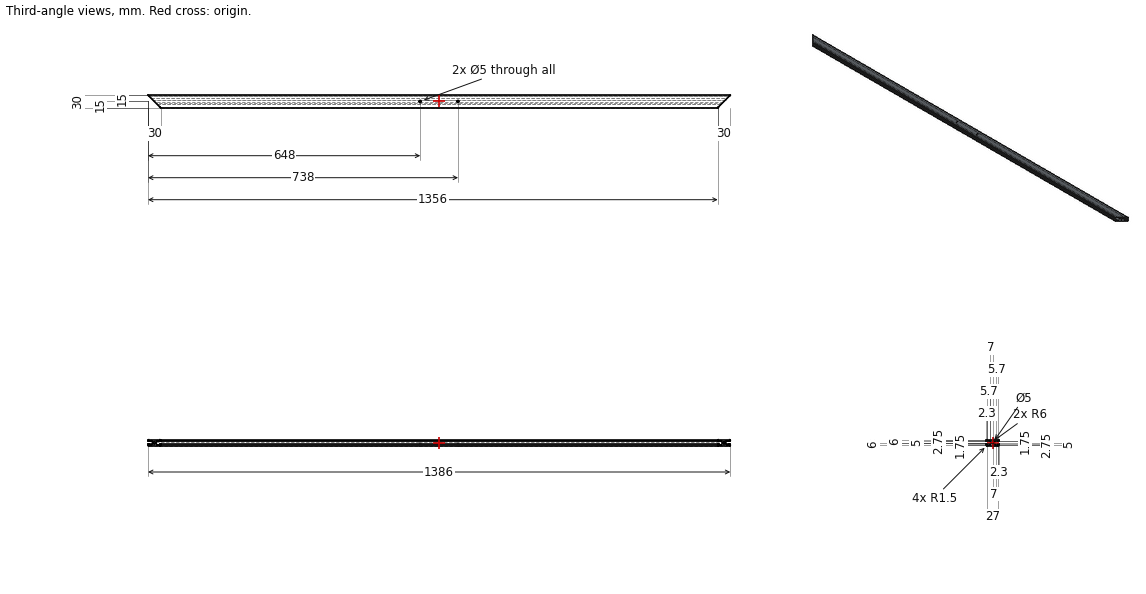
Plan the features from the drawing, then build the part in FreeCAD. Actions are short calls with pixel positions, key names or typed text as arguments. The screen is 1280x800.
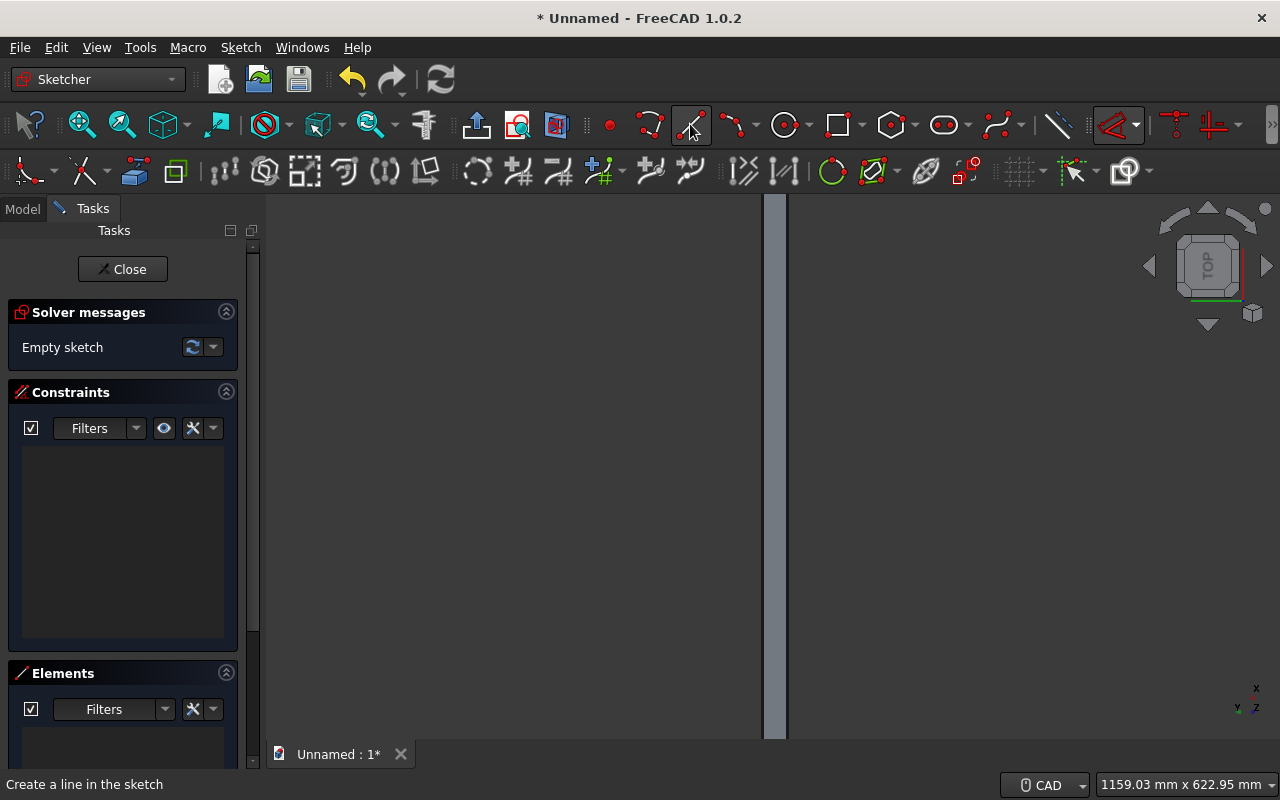
scroll(674, 467, down, 6)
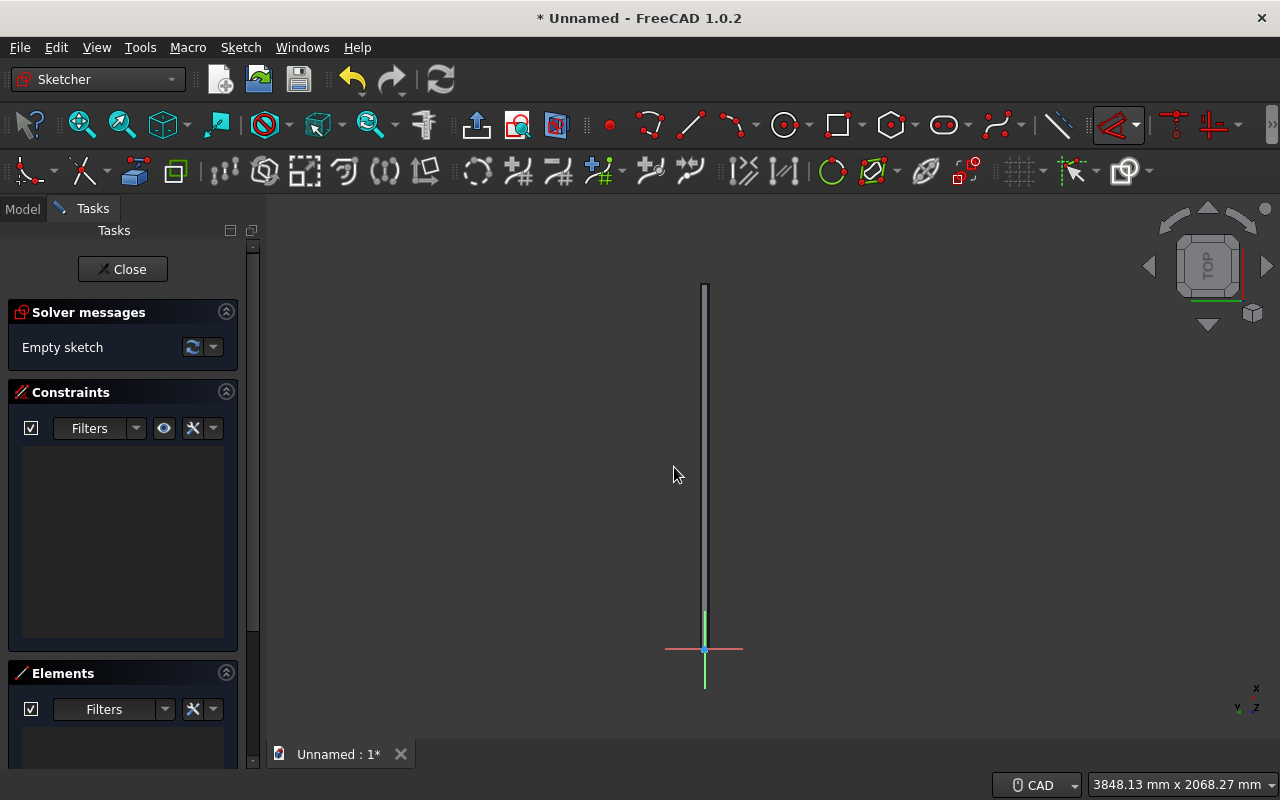
click(650, 126)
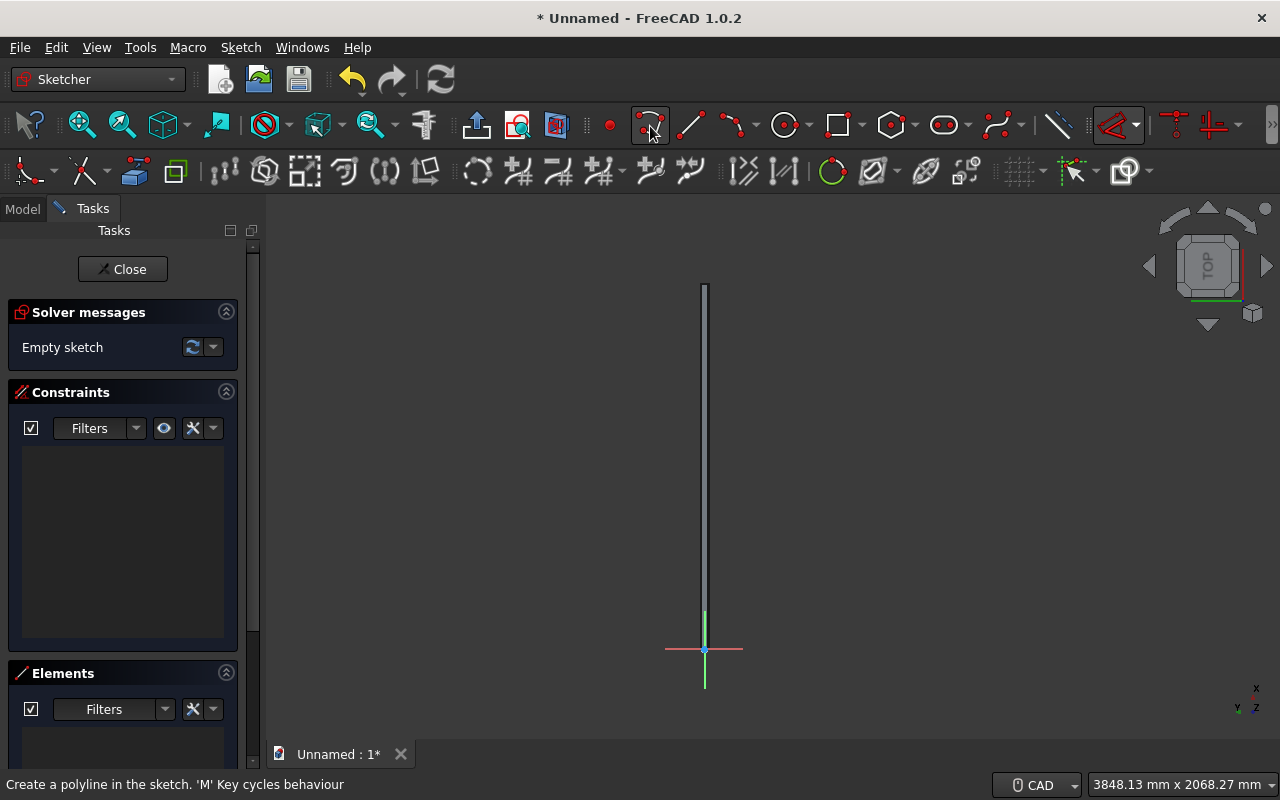
scroll(701, 649, up, 7)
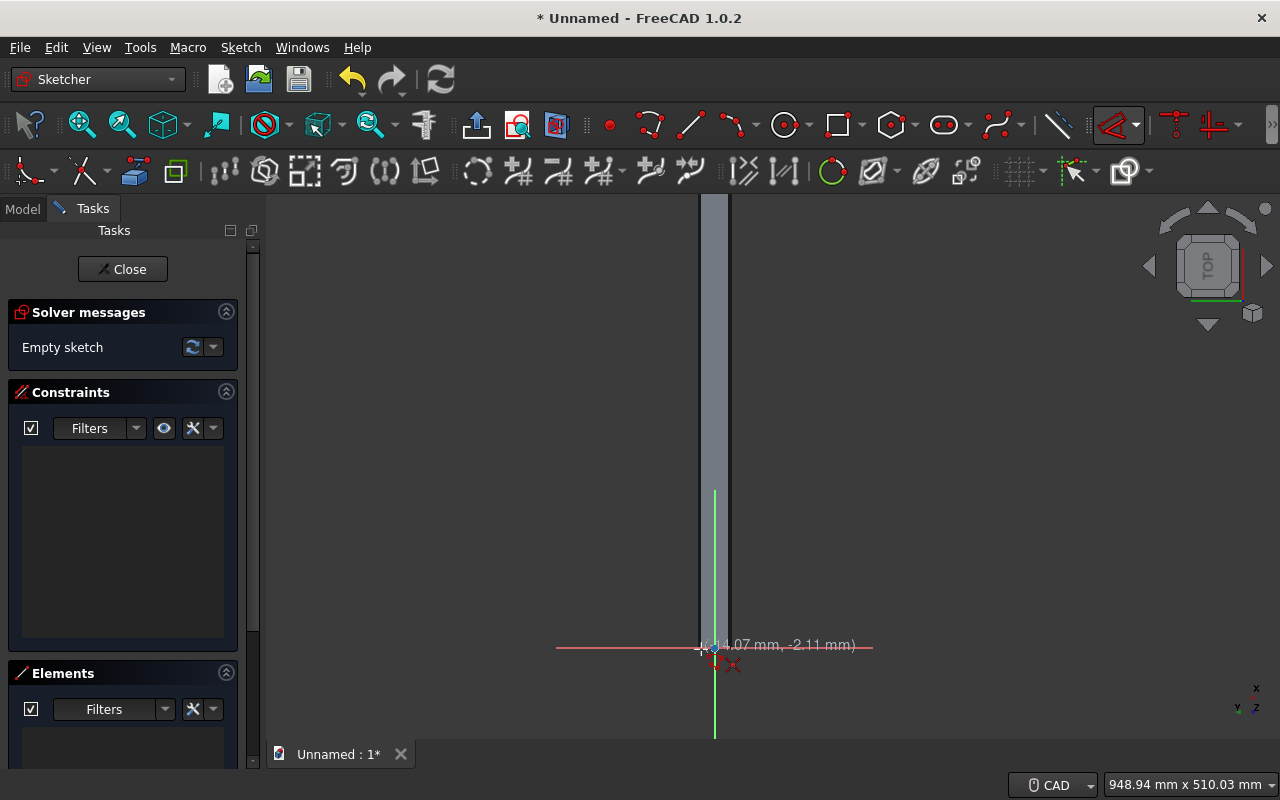
click(699, 648)
click(731, 639)
click(731, 616)
click(699, 648)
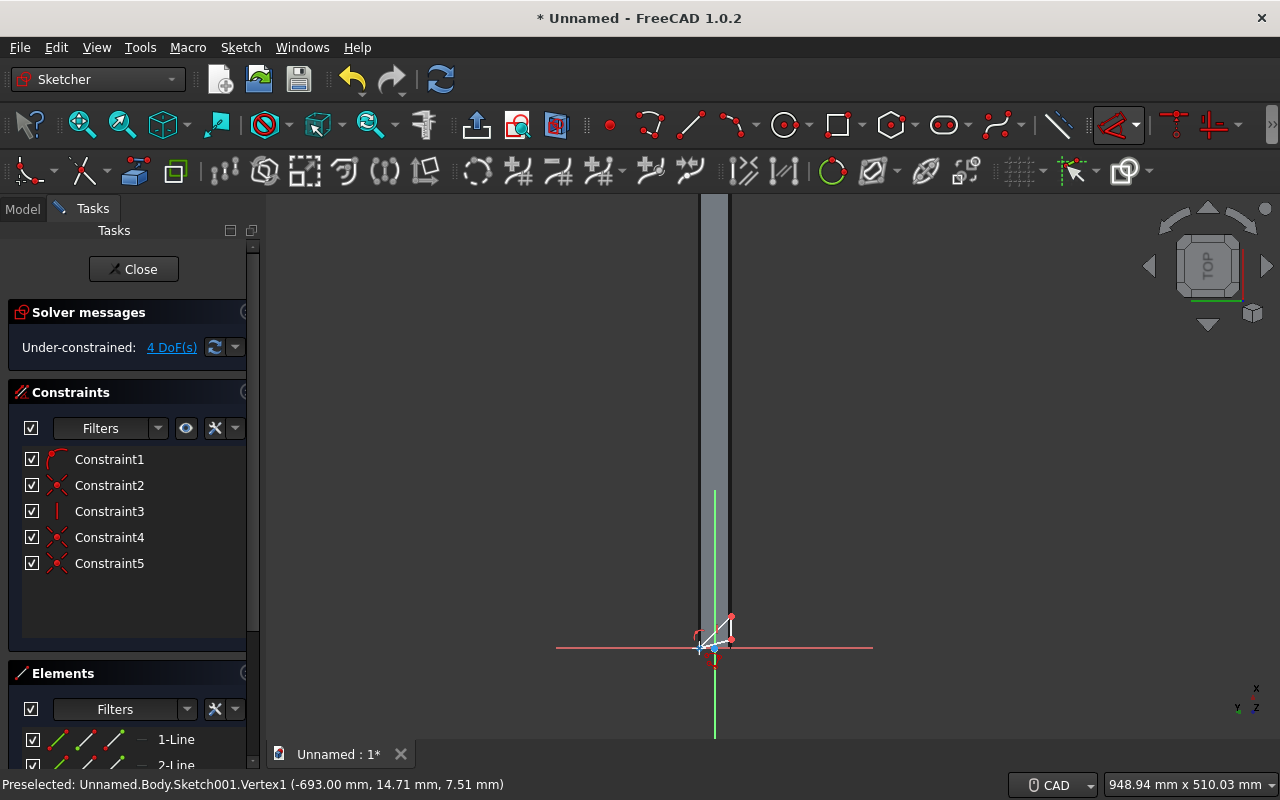
scroll(701, 649, down, 7)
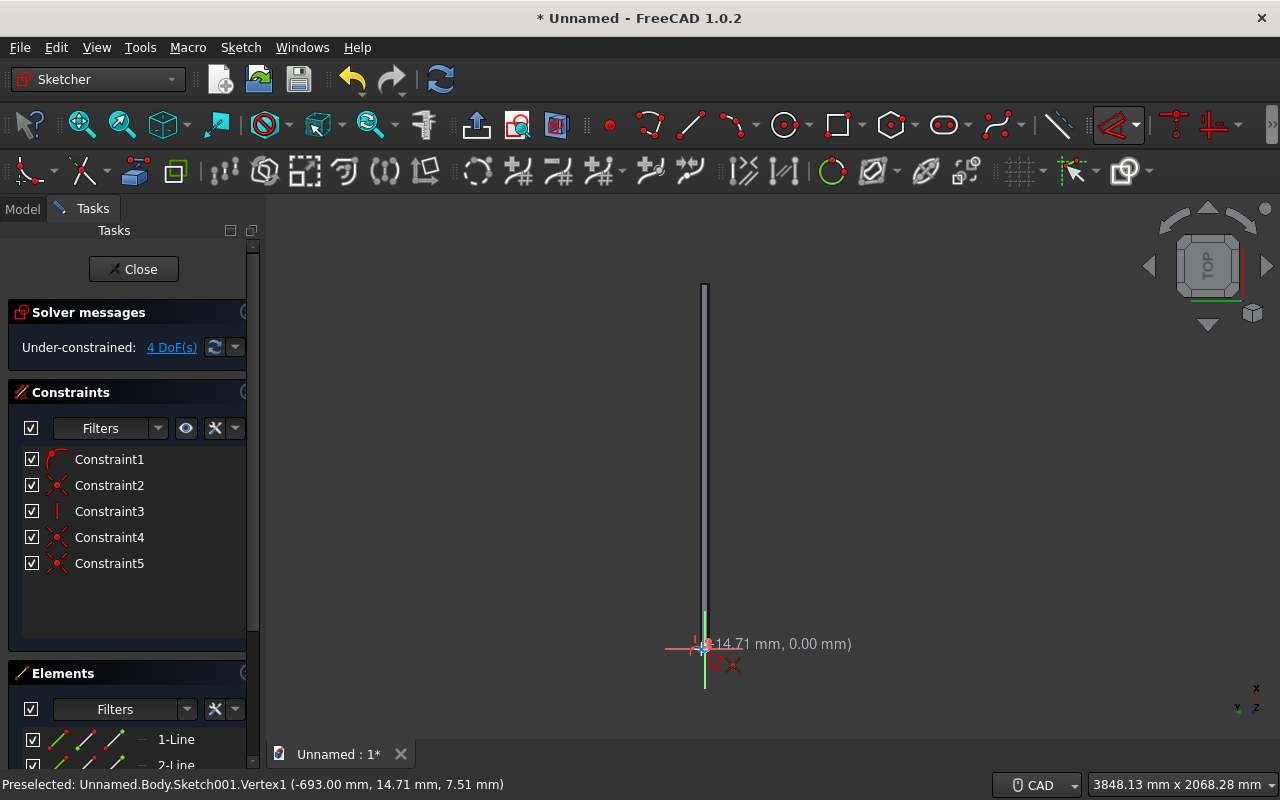
scroll(709, 292, up, 7)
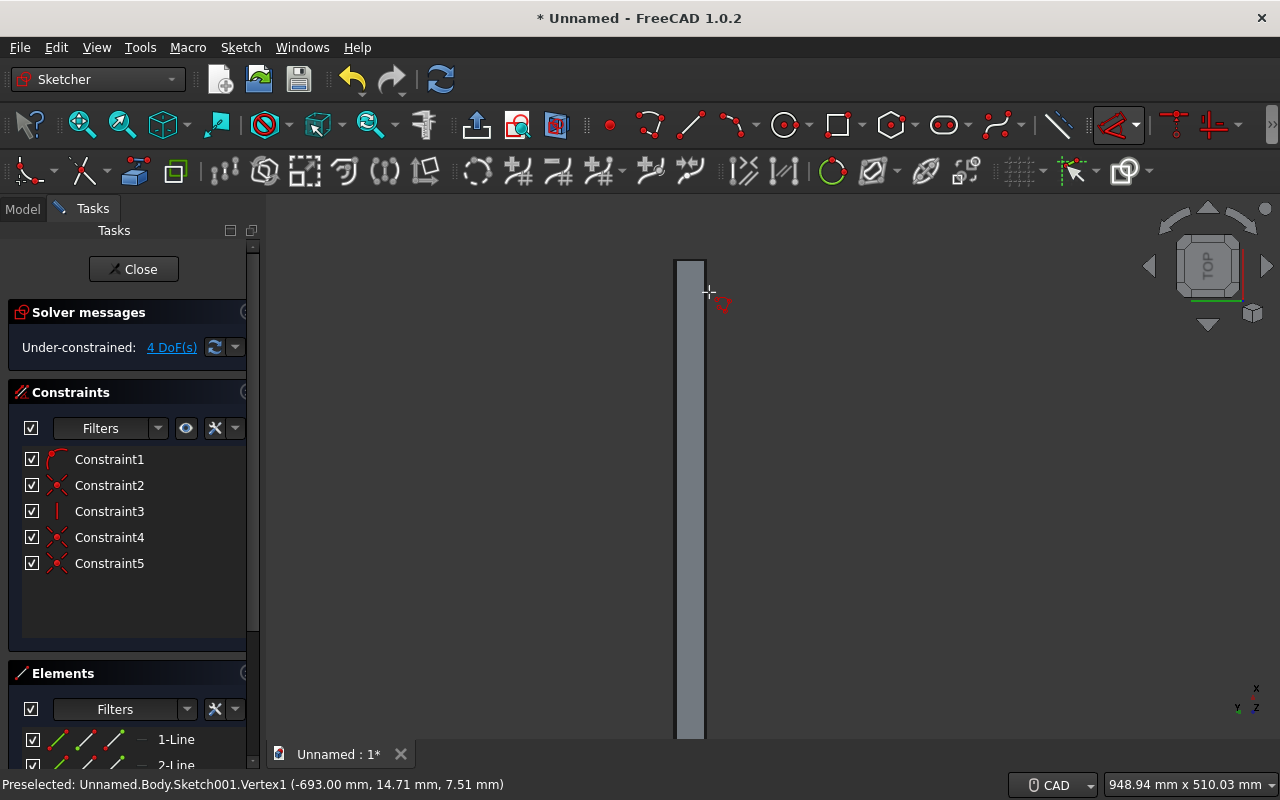
click(706, 292)
click(706, 260)
click(674, 260)
click(706, 293)
key(Escape)
key(Escape)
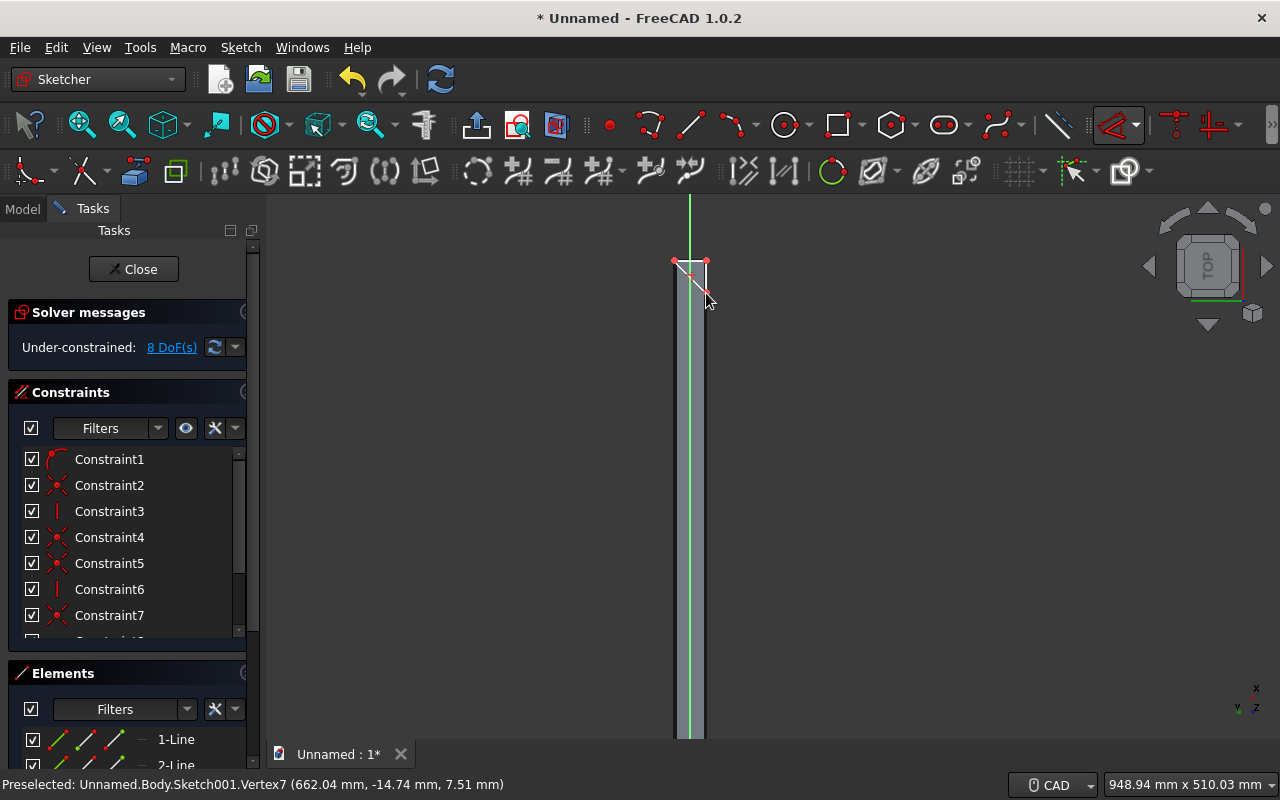
scroll(709, 292, down, 7)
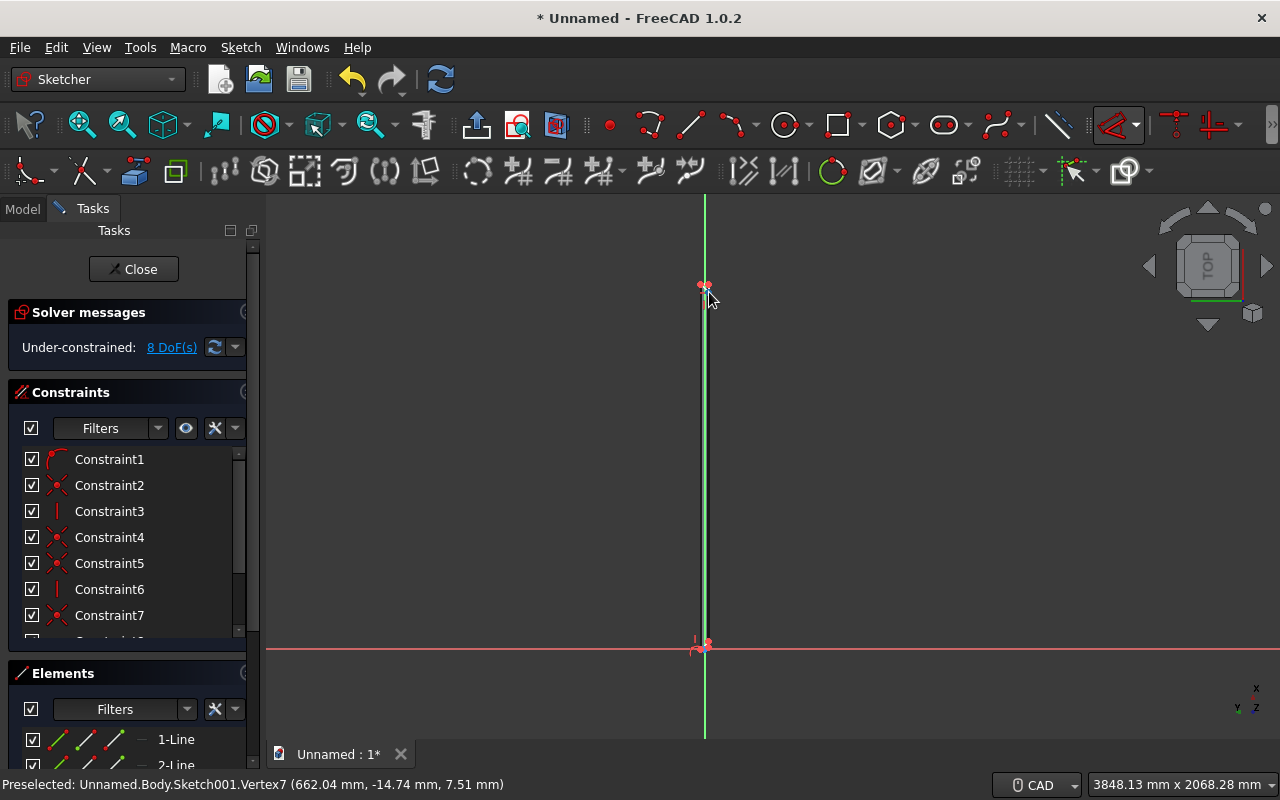
scroll(707, 648, up, 11)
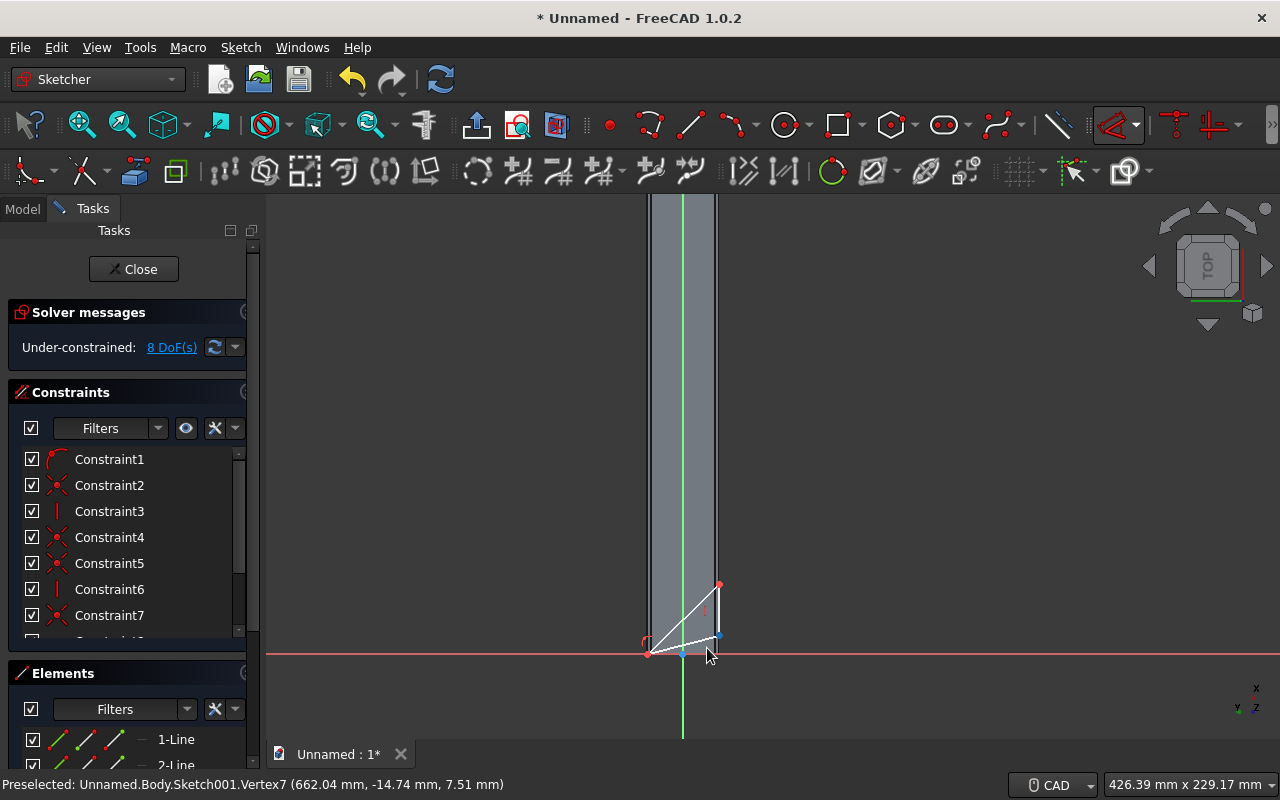
click(705, 640)